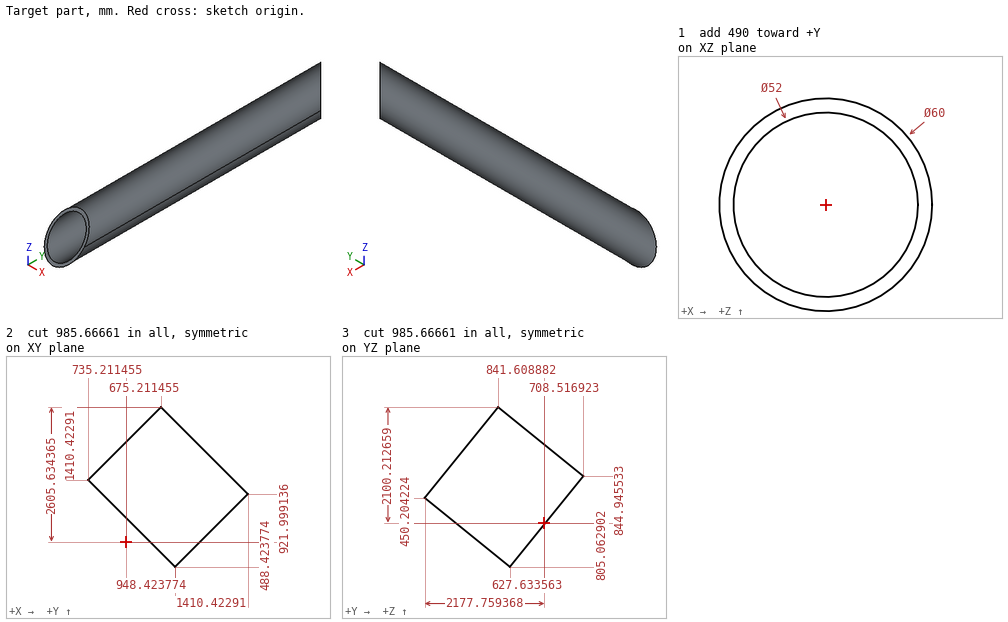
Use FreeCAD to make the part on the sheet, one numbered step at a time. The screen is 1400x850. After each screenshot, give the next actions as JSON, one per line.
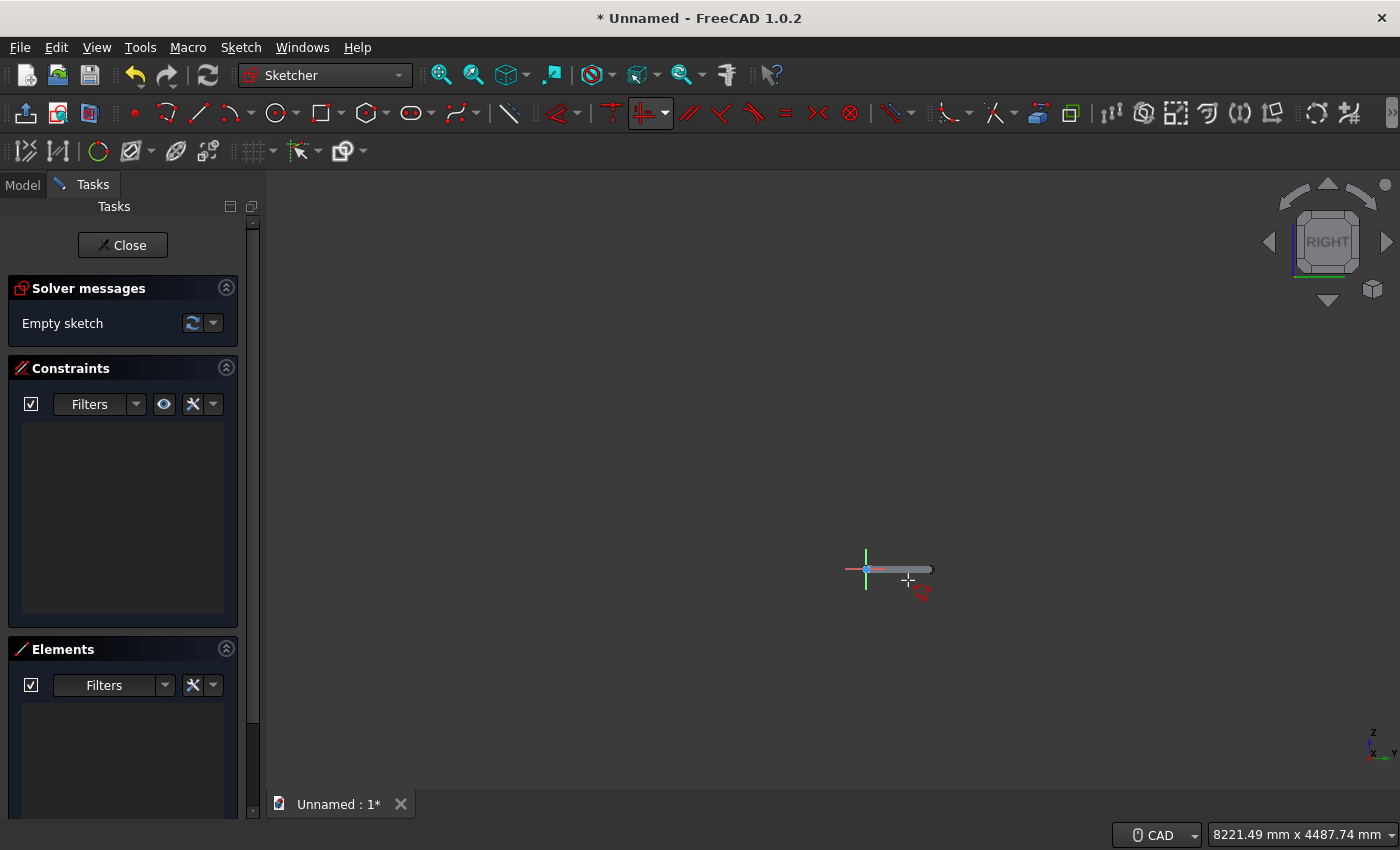
{"action": "left_click", "coordinate": [780, 680]}
{"action": "left_click", "coordinate": [964, 453]}
{"action": "left_click", "coordinate": [750, 280]}
{"action": "left_click", "coordinate": [566, 507]}
{"action": "left_click", "coordinate": [780, 681]}
{"action": "key", "text": "Escape"}
{"action": "key", "text": "Escape"}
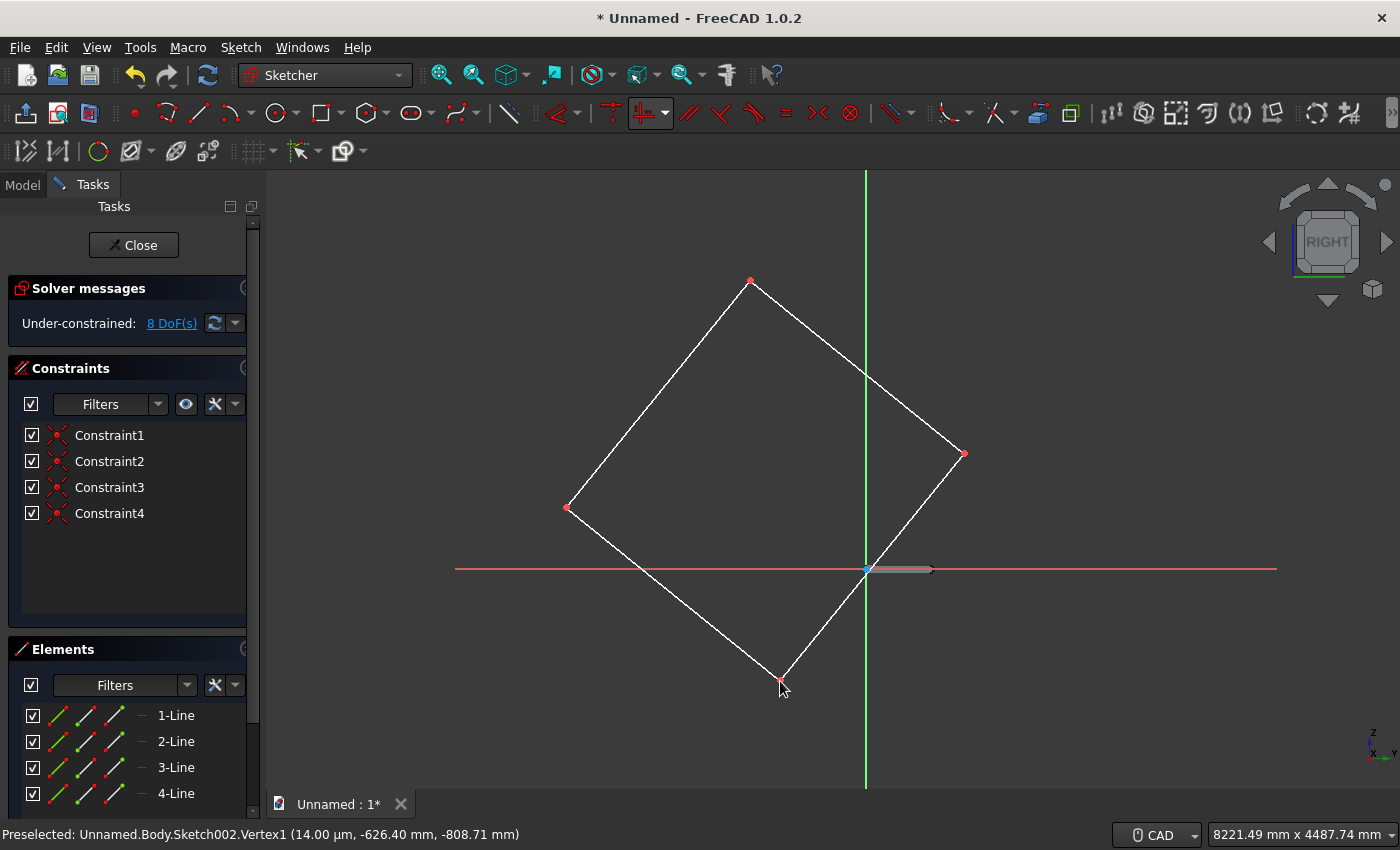
{"action": "key", "text": "d"}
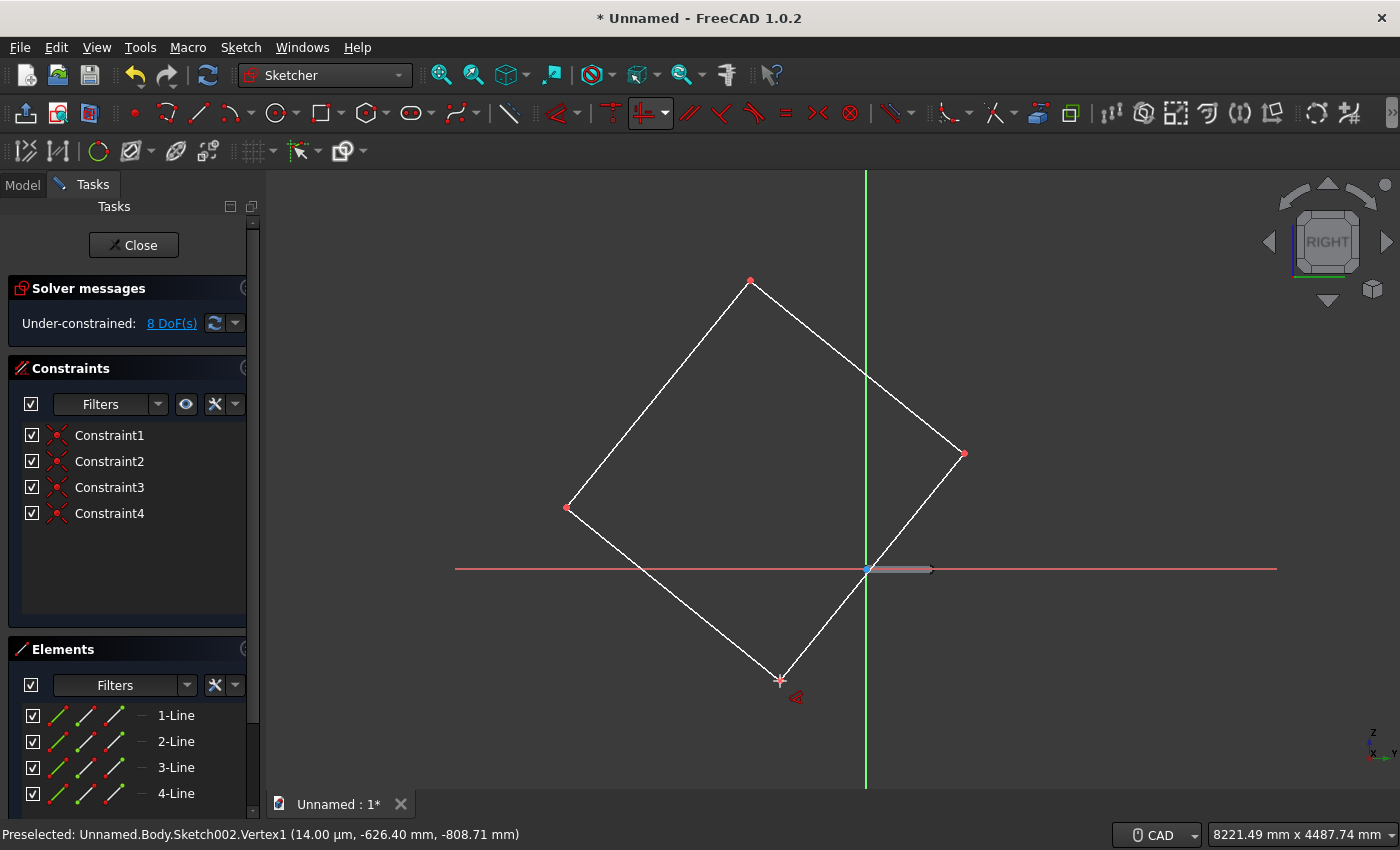
{"action": "left_click", "coordinate": [780, 681]}
{"action": "left_click", "coordinate": [823, 715]}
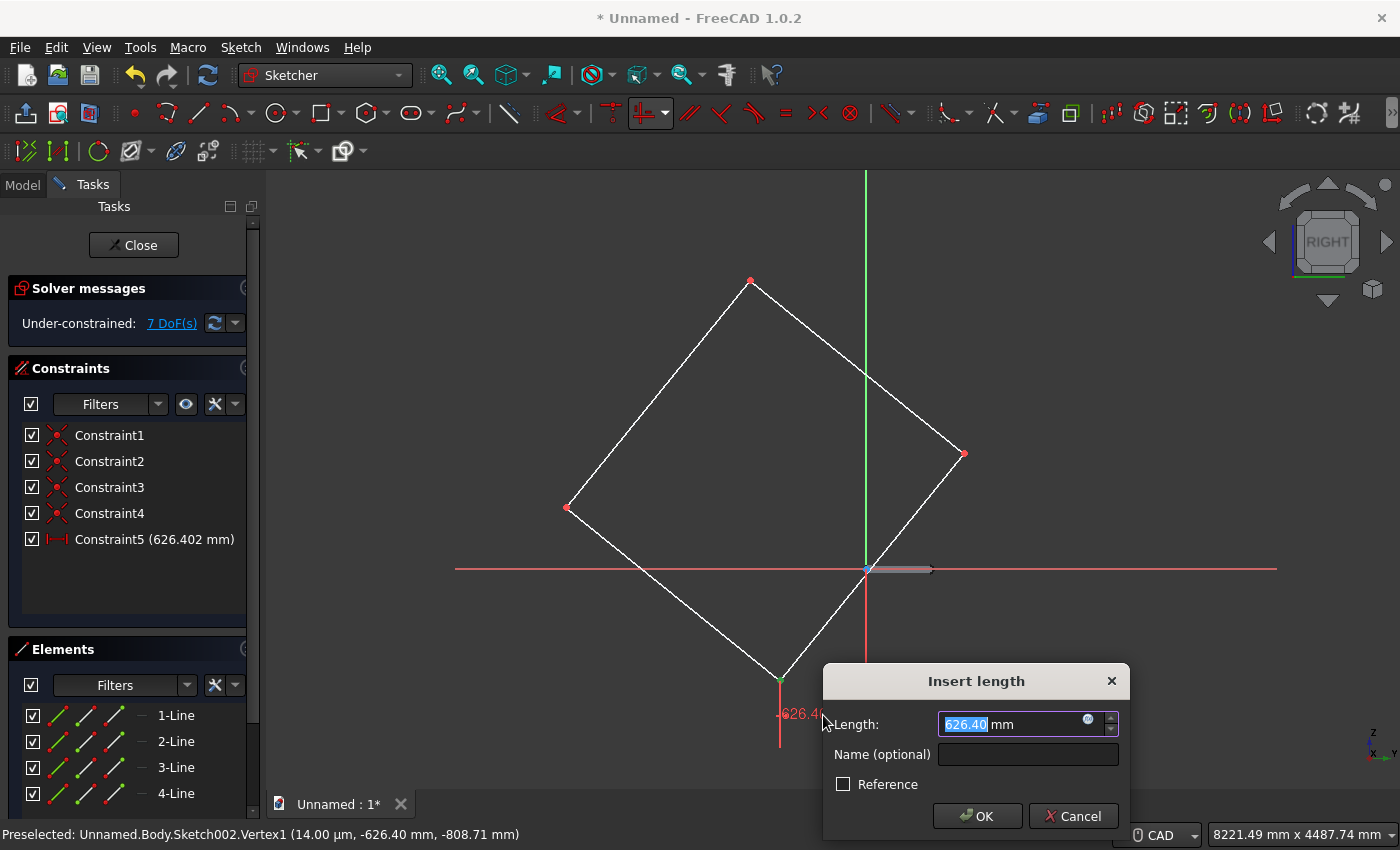
{"action": "type", "text": "627.633563"}
{"action": "key", "text": "Return"}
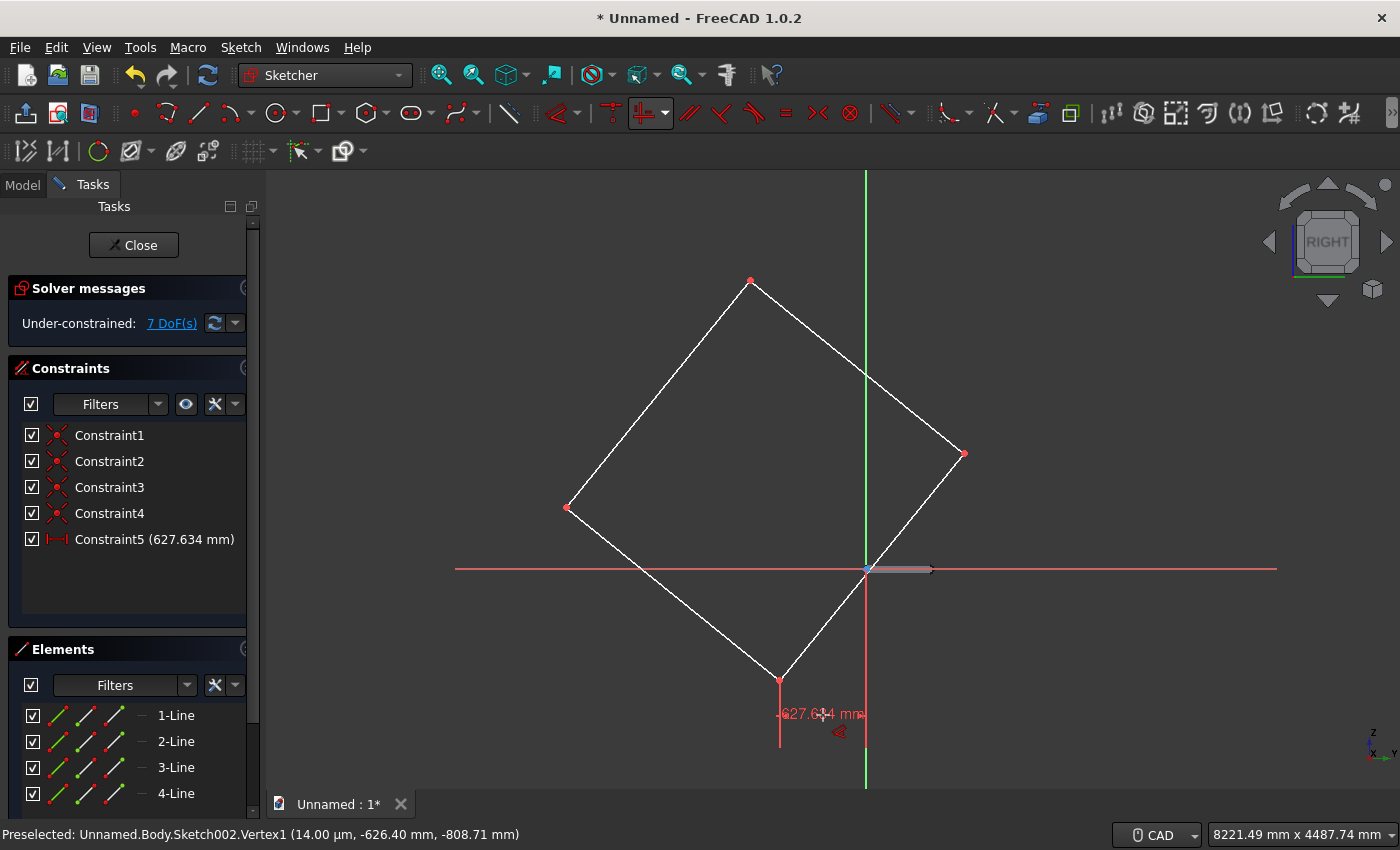
{"action": "left_click", "coordinate": [780, 681]}
{"action": "left_click", "coordinate": [900, 625]}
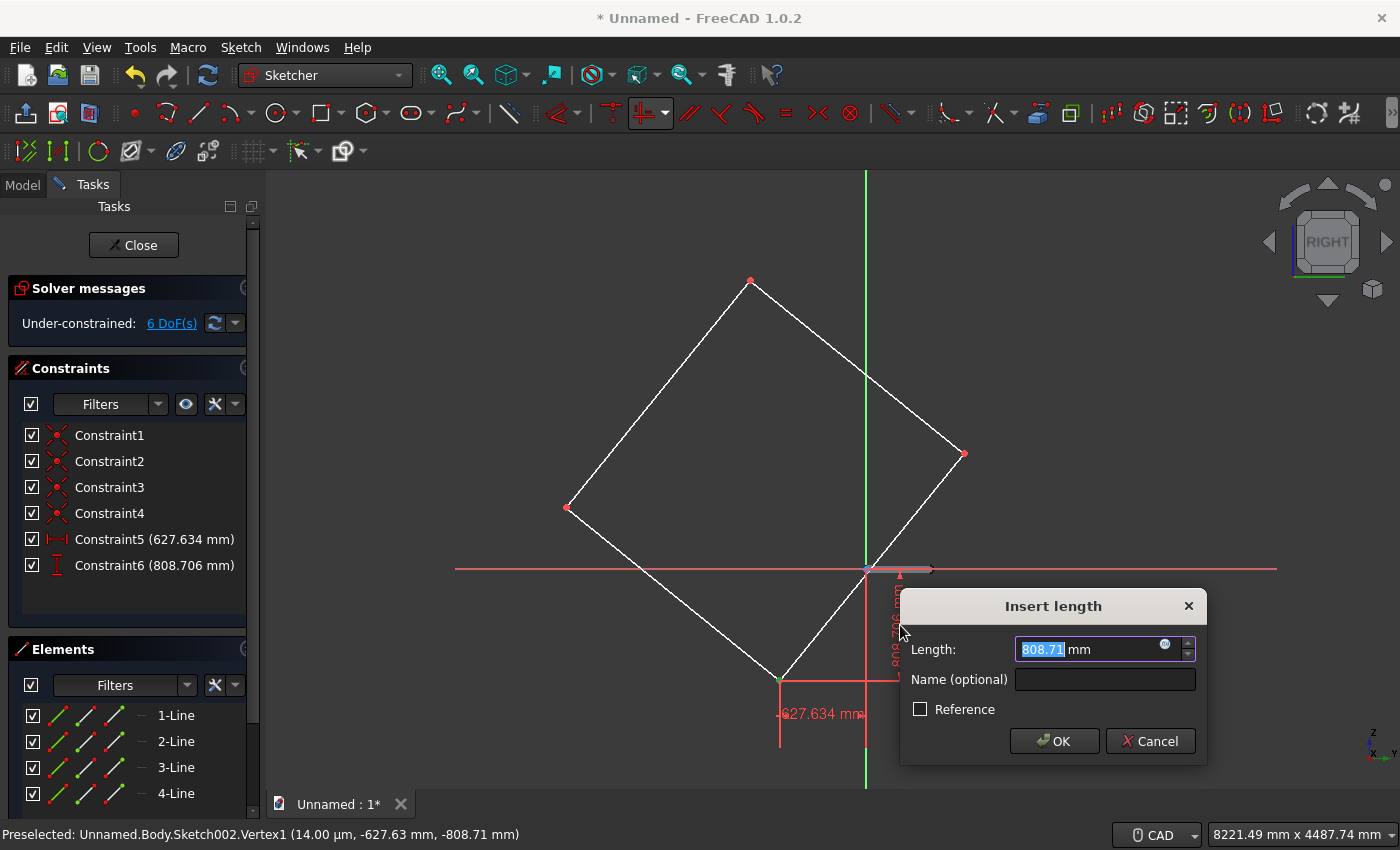
{"action": "type", "text": "805.062902"}
{"action": "key", "text": "Return"}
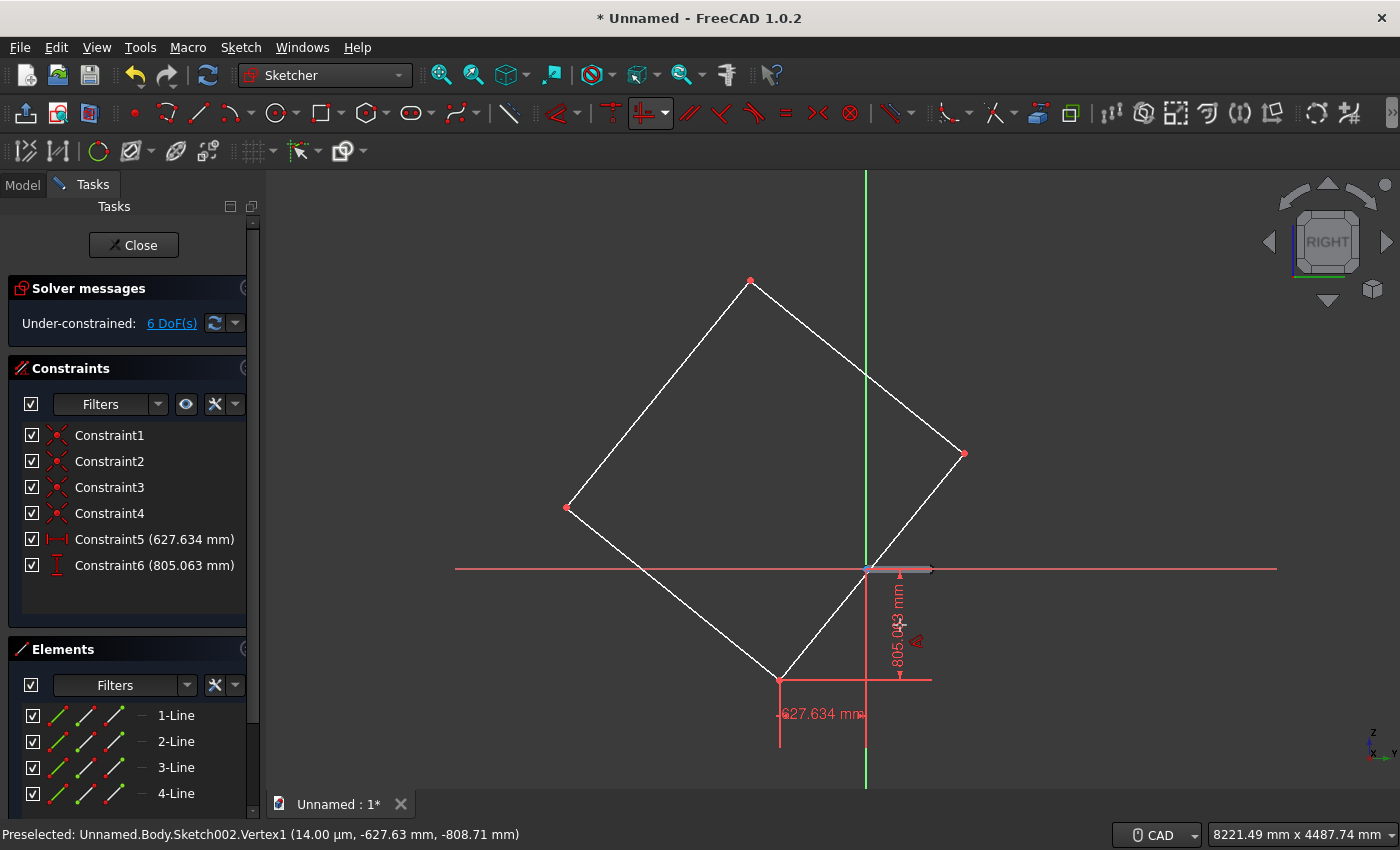
{"action": "left_click", "coordinate": [964, 454]}
{"action": "left_click", "coordinate": [915, 603]}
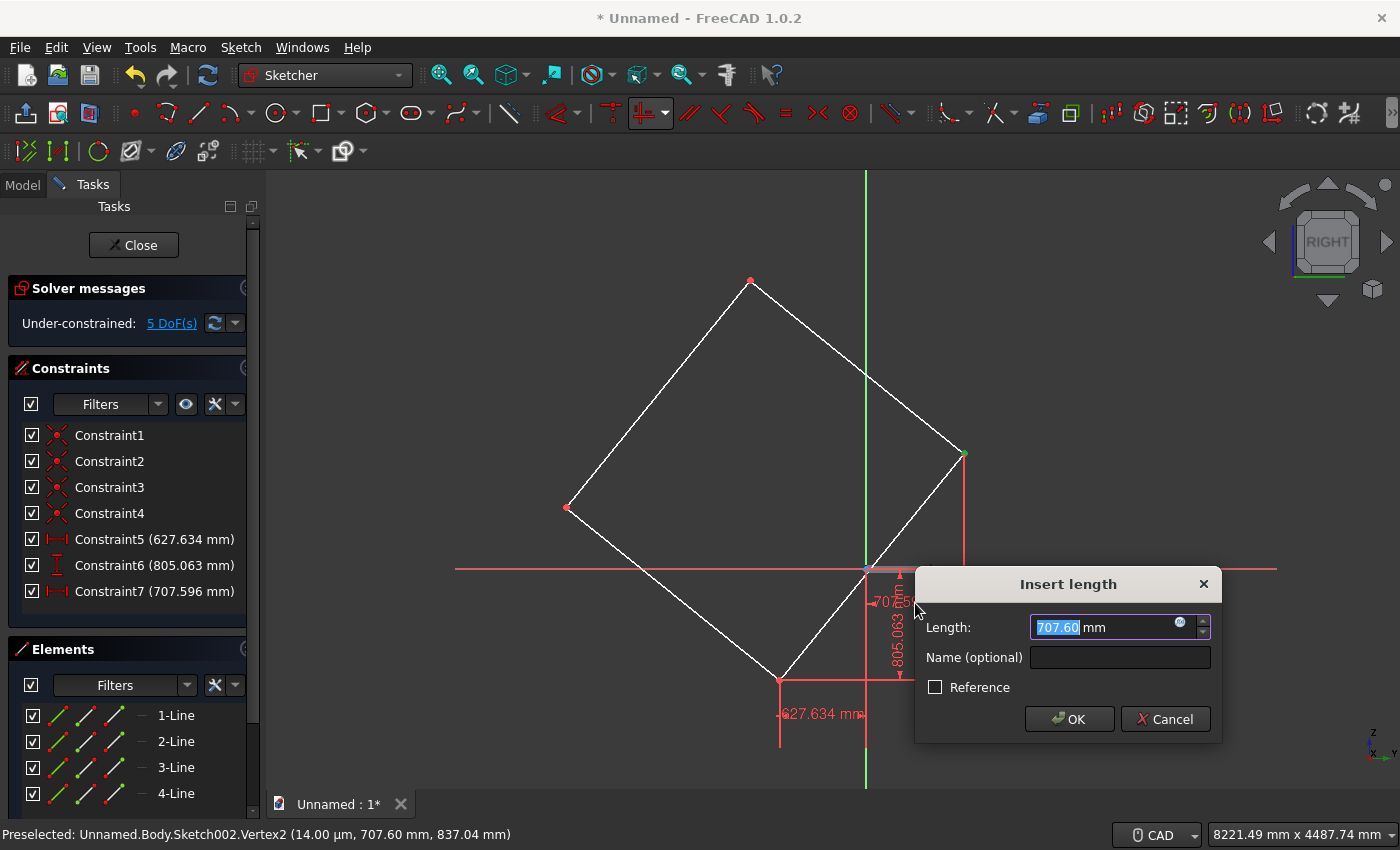
{"action": "type", "text": "708.516923"}
{"action": "key", "text": "Return"}